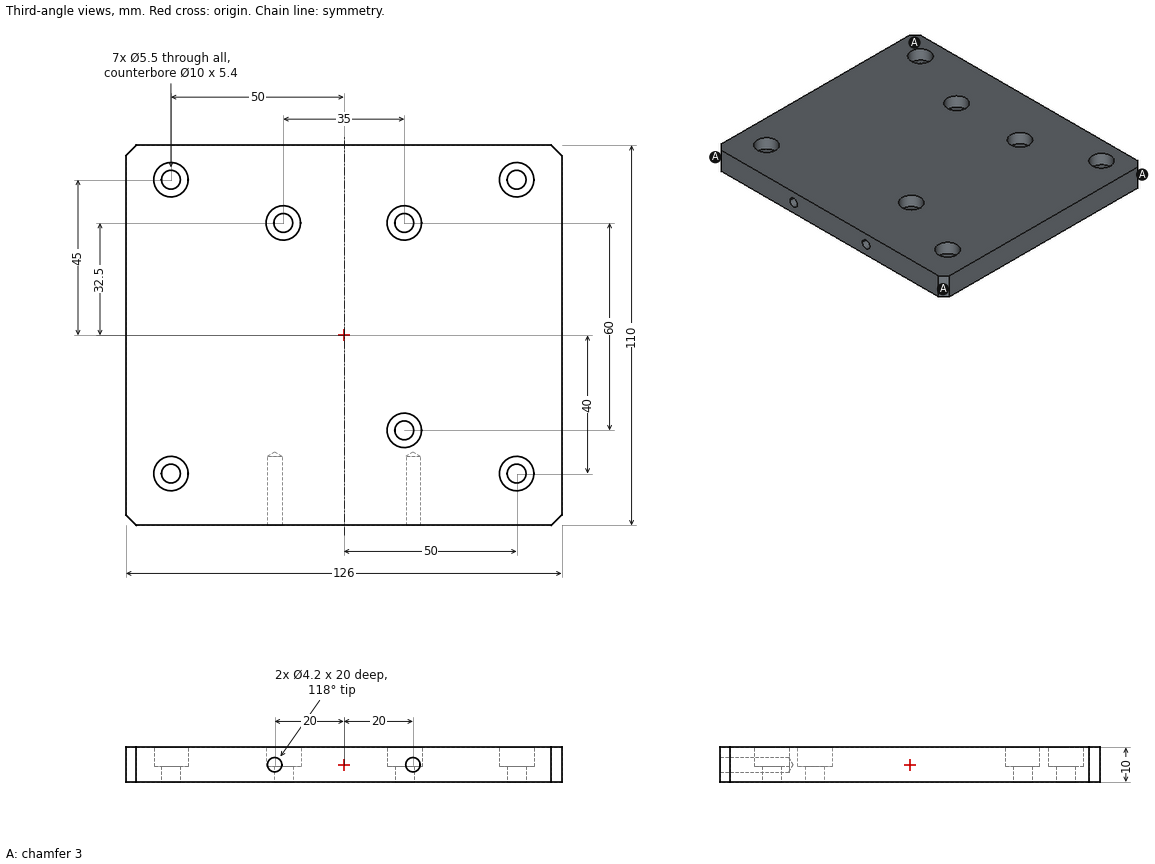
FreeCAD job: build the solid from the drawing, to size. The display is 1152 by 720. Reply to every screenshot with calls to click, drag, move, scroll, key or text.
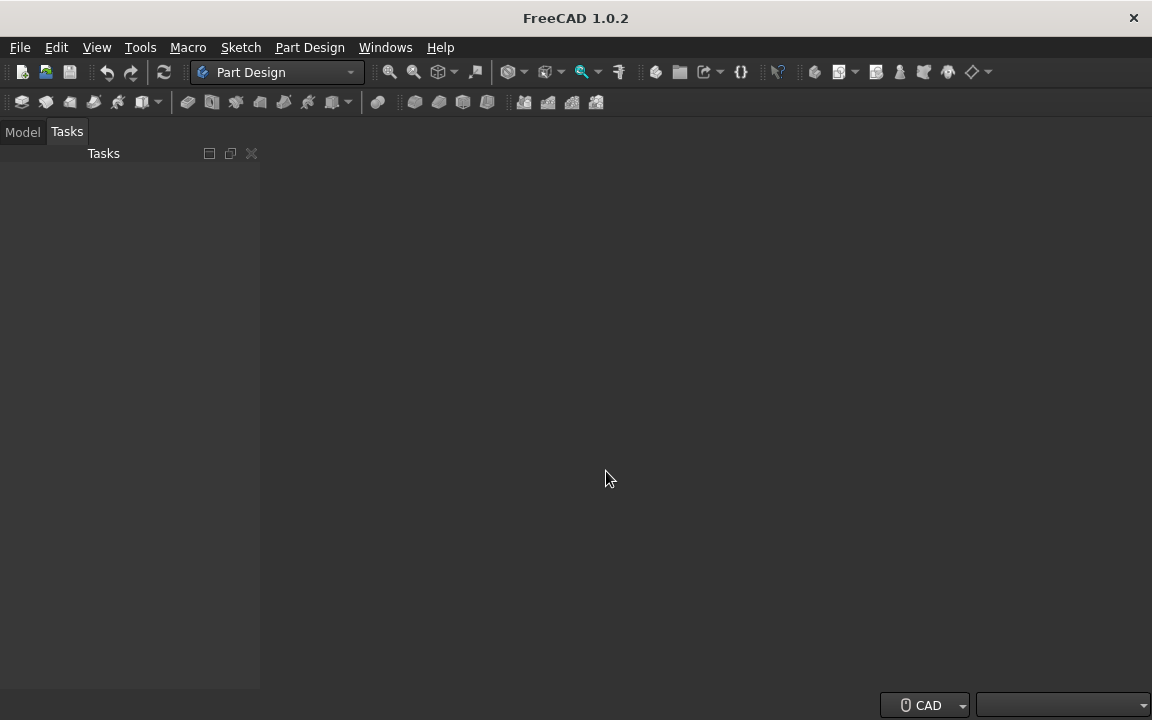
click(22, 72)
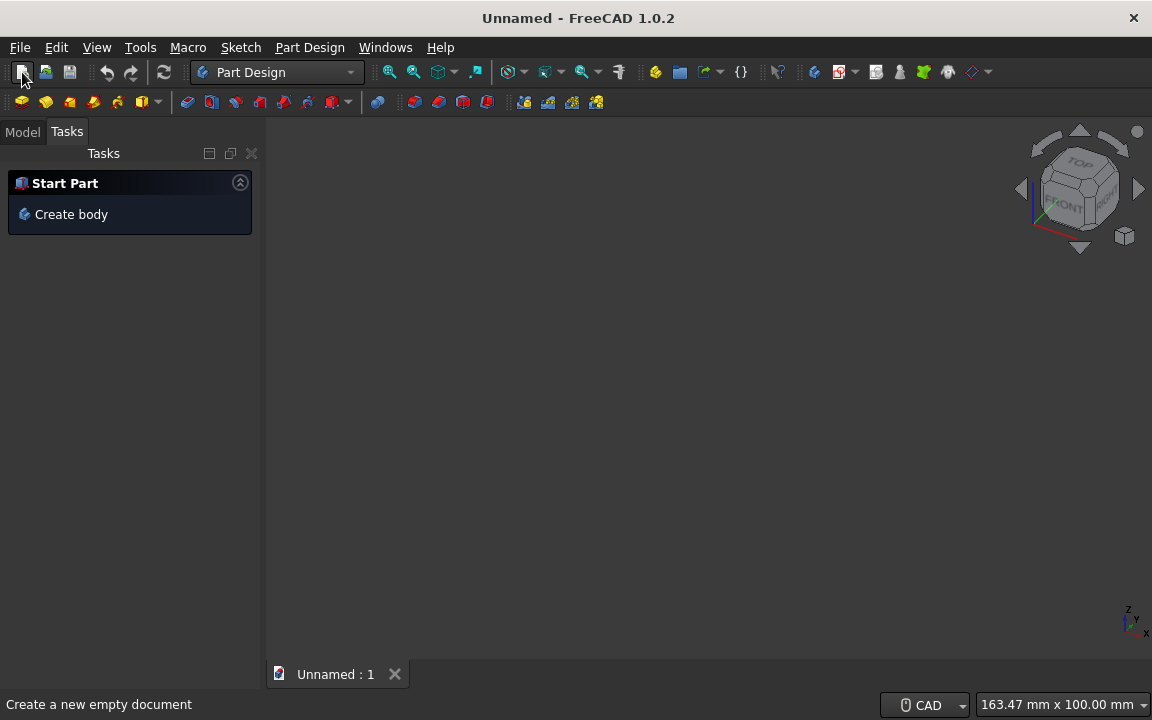
click(840, 72)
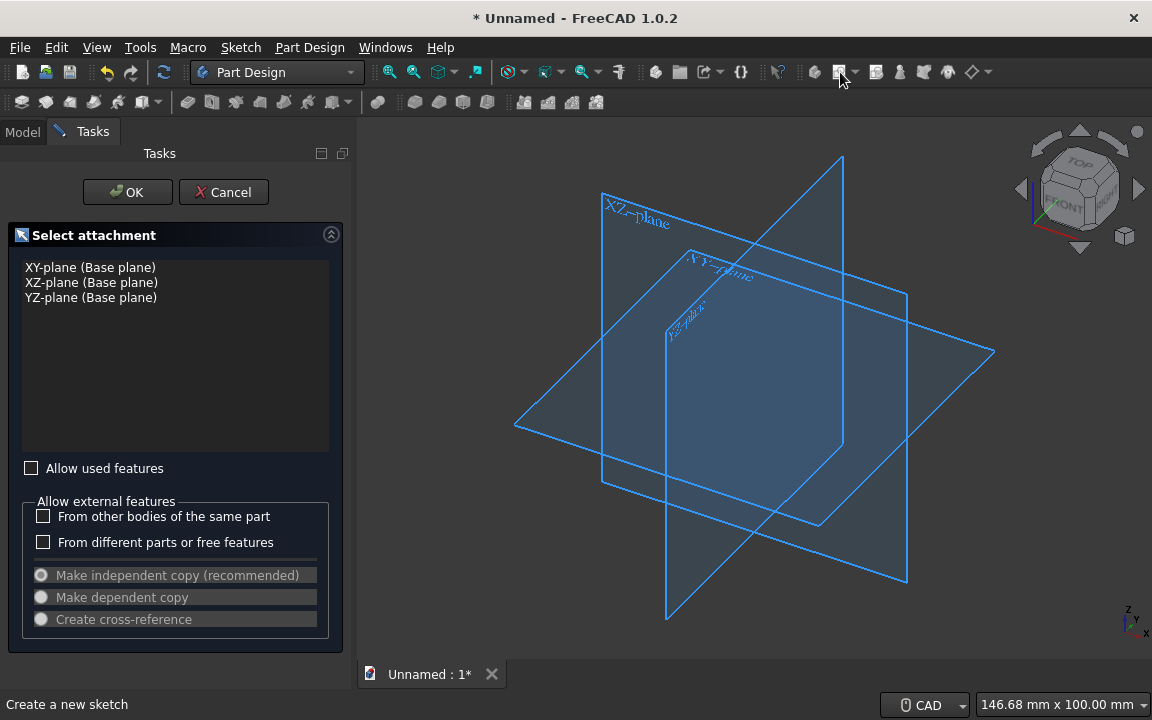
click(82, 268)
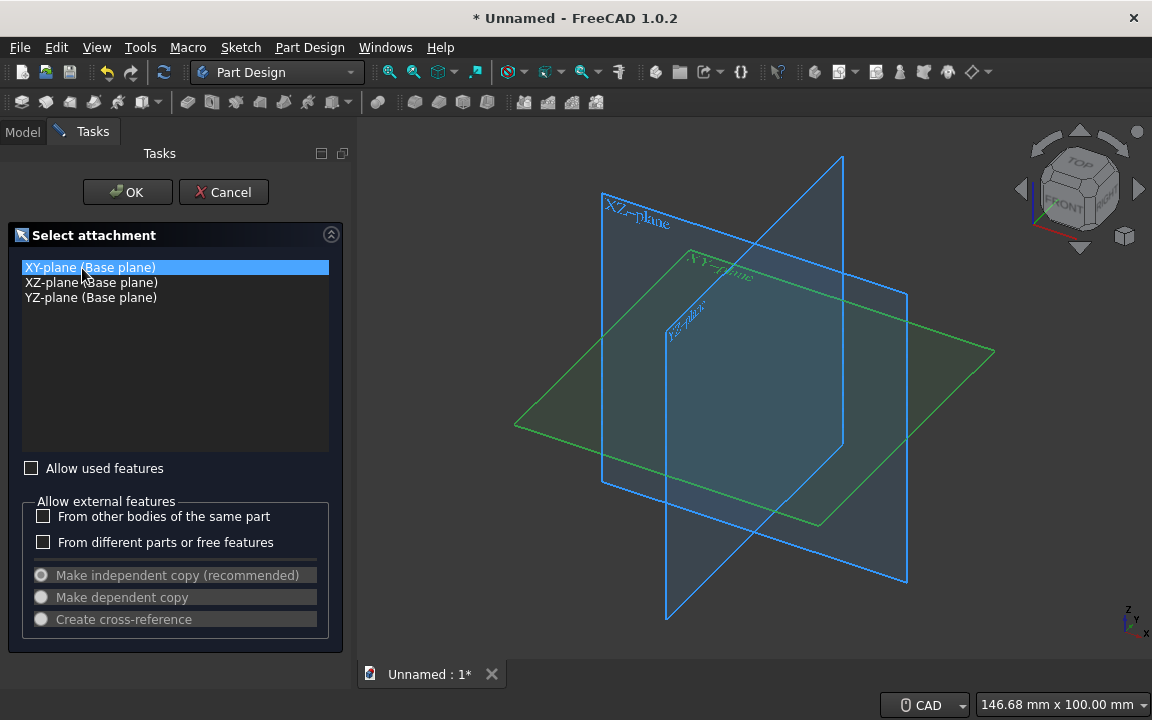
click(128, 192)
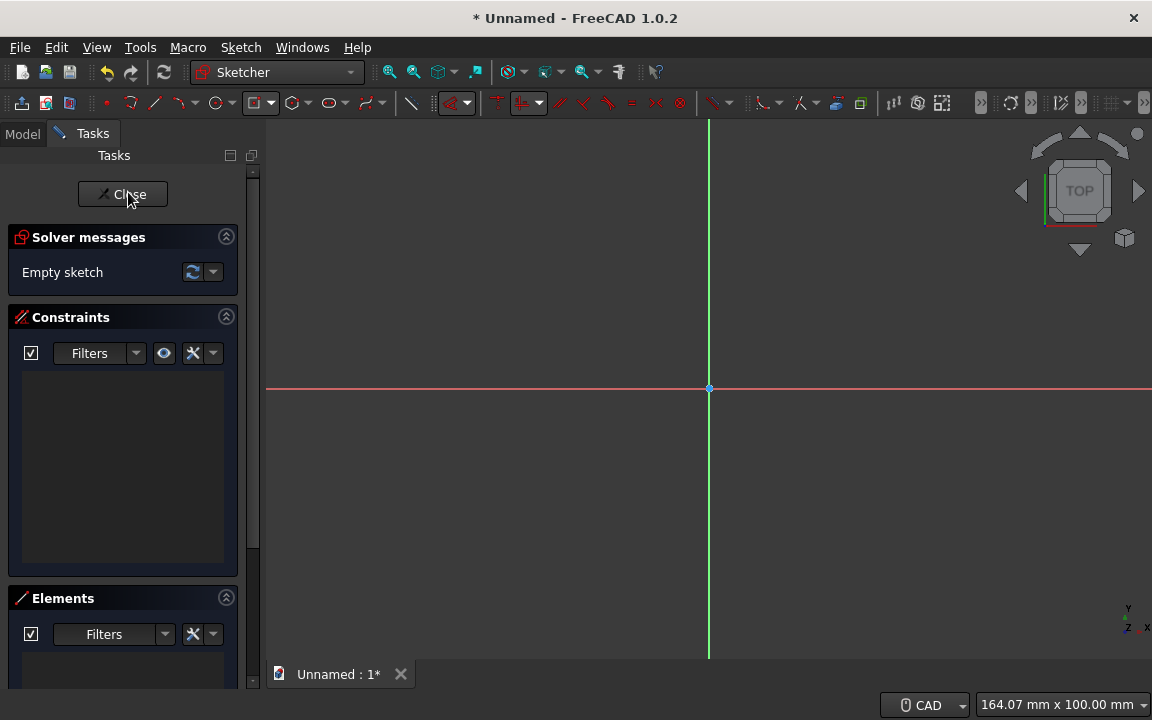
scroll(557, 389, down, 3)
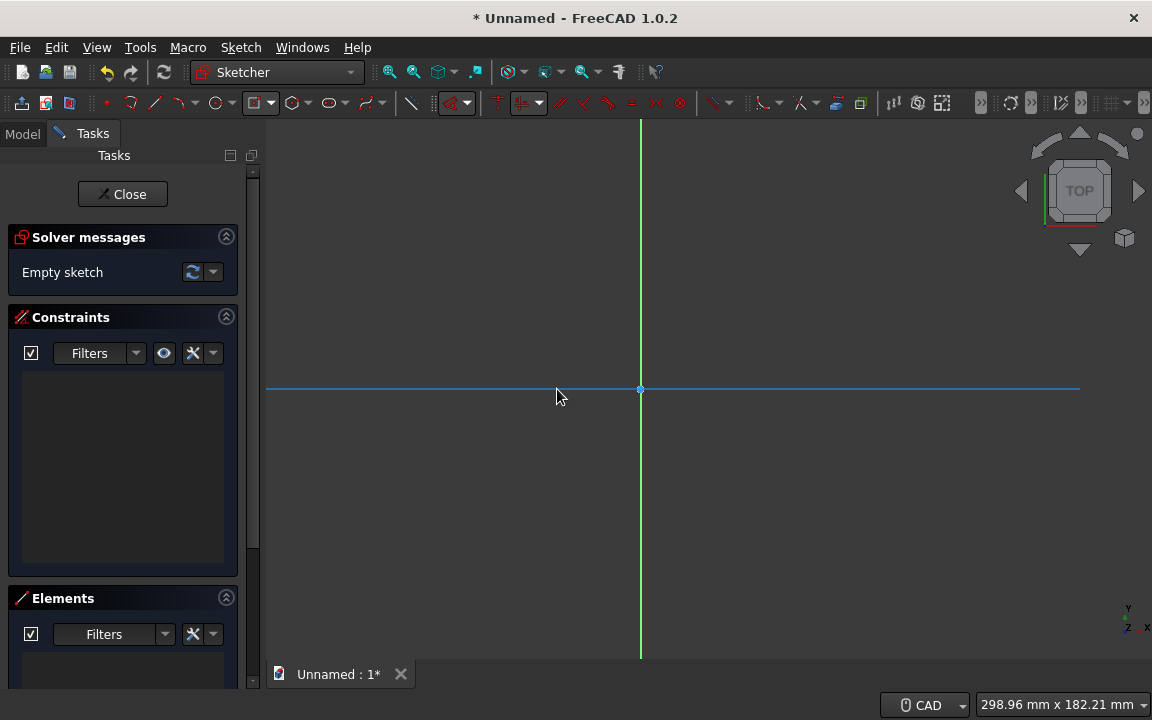
click(254, 104)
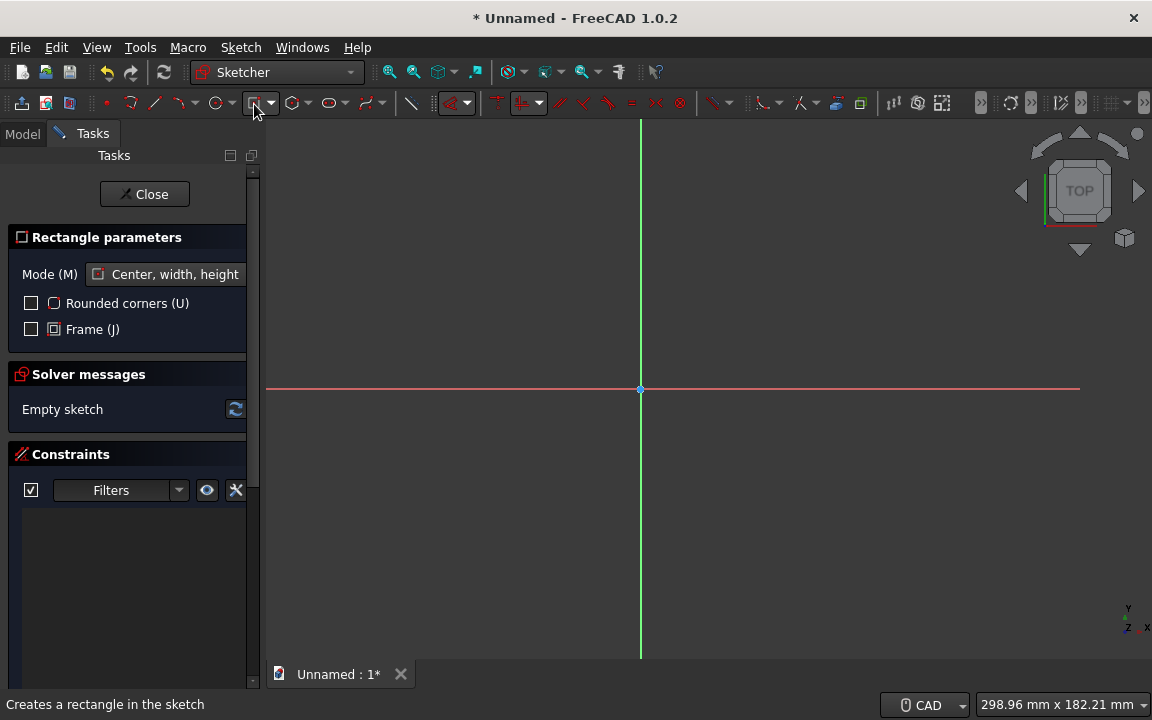
click(641, 389)
move(827, 226)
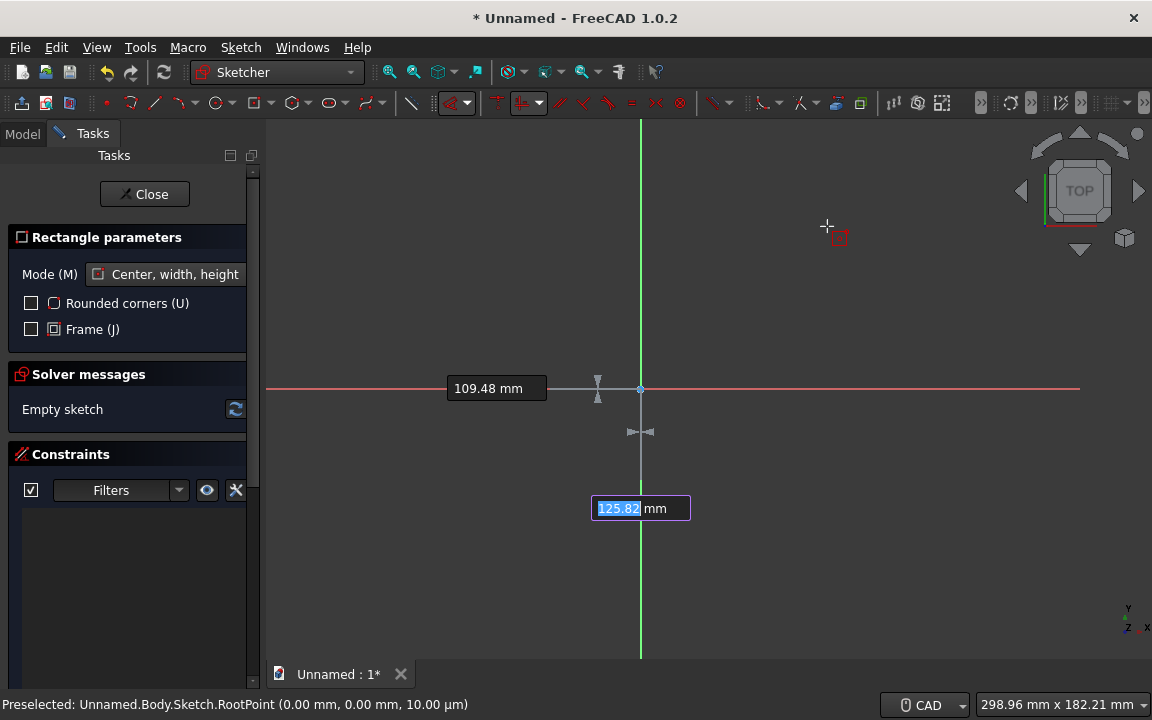
text(126)
key(Tab)
text(110)
key(Return)
key(Escape)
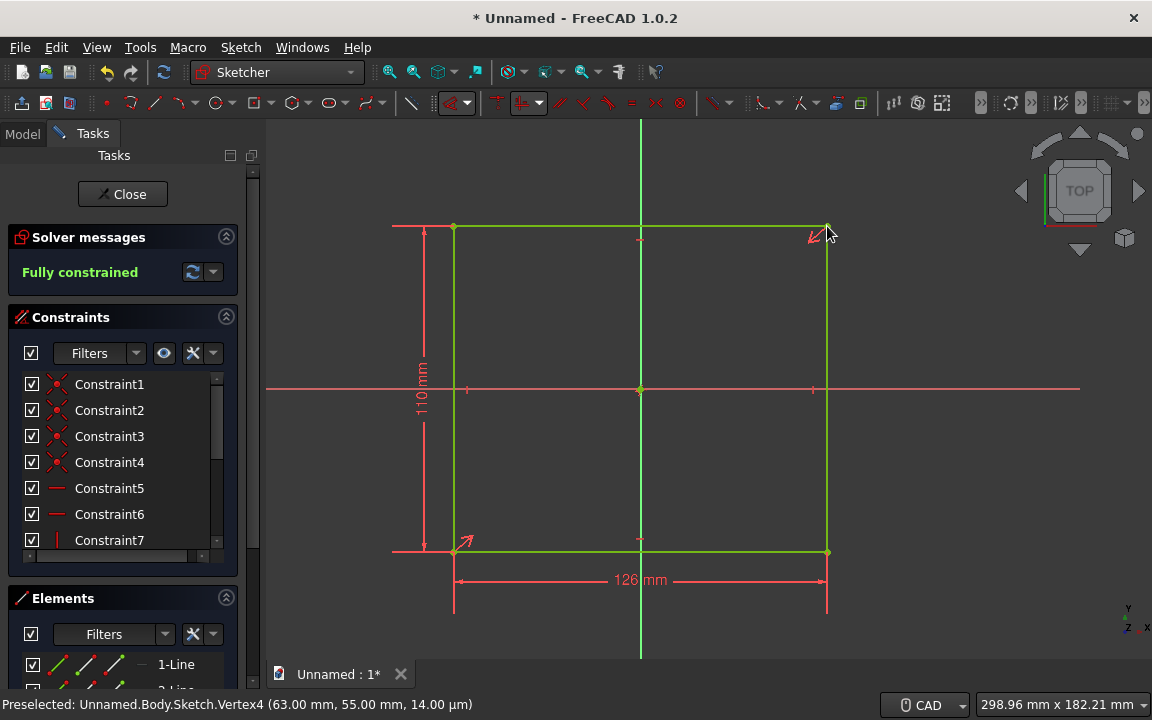
click(123, 194)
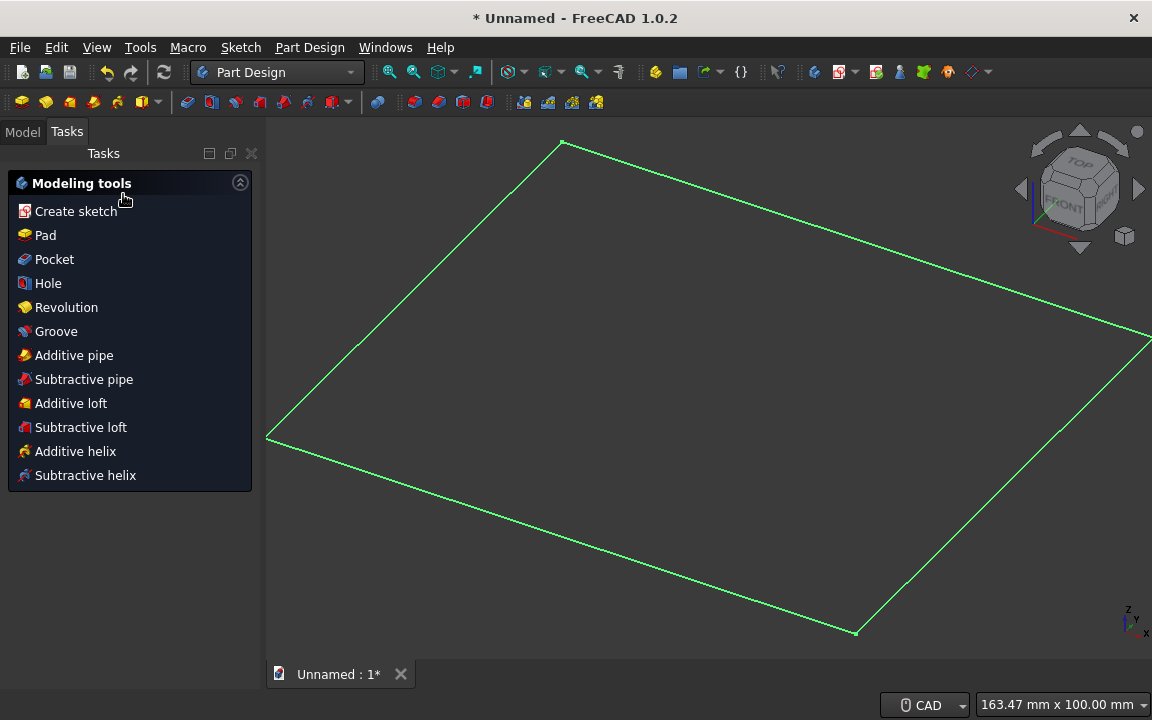
click(22, 102)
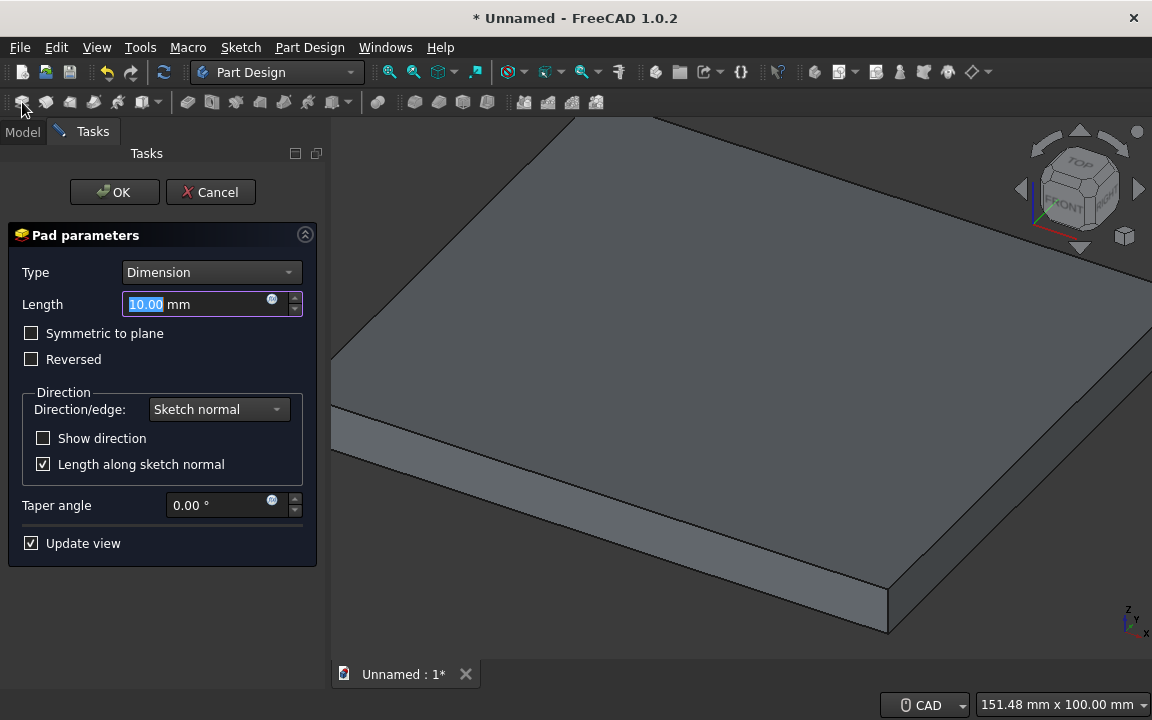
text(10)
key(Tab)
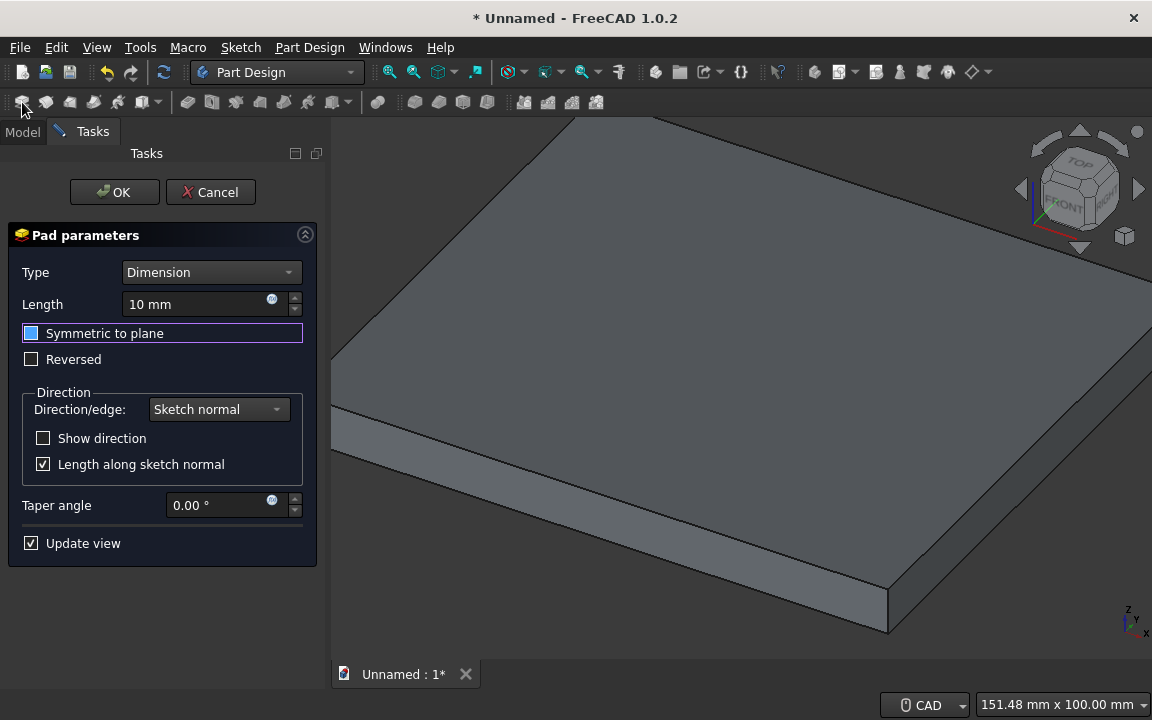
click(30, 333)